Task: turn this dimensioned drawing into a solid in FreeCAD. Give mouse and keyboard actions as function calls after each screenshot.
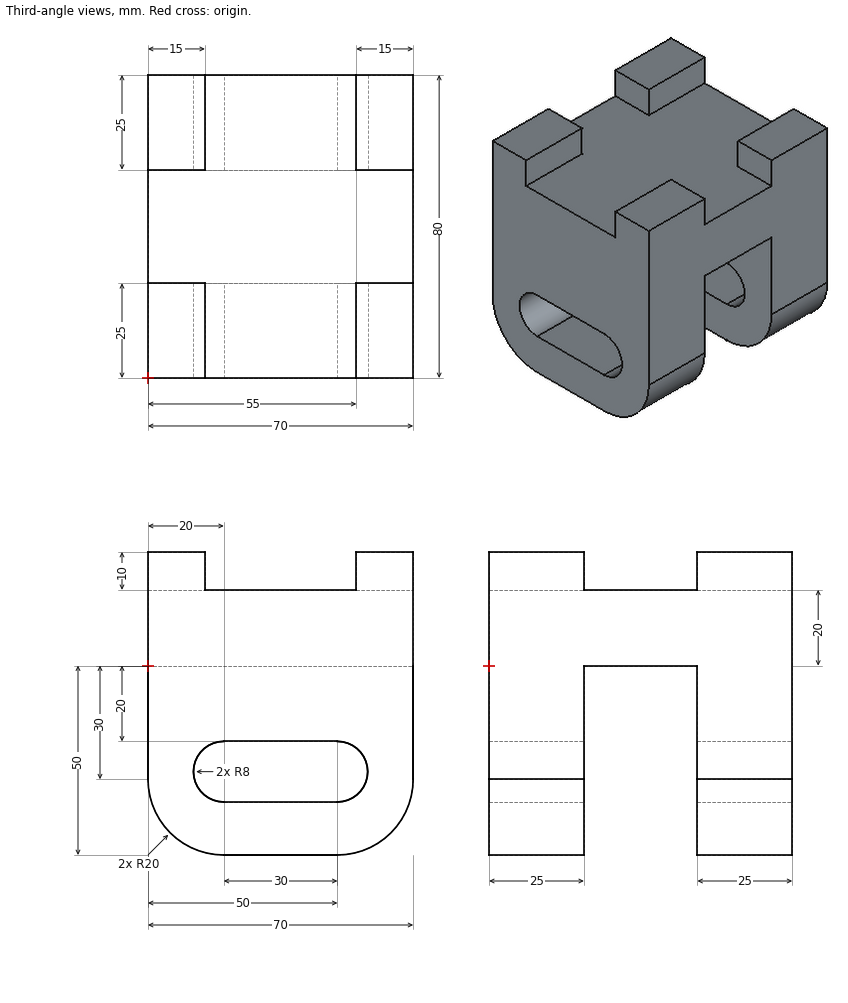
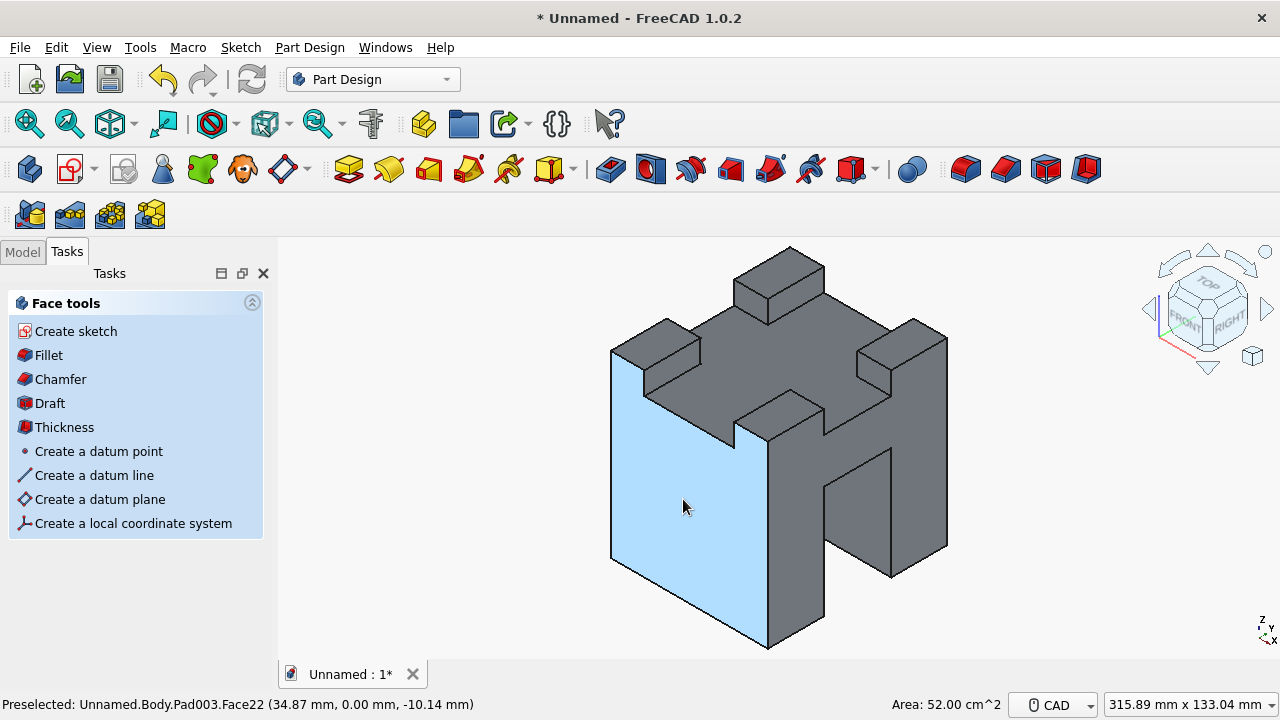
click(70, 170)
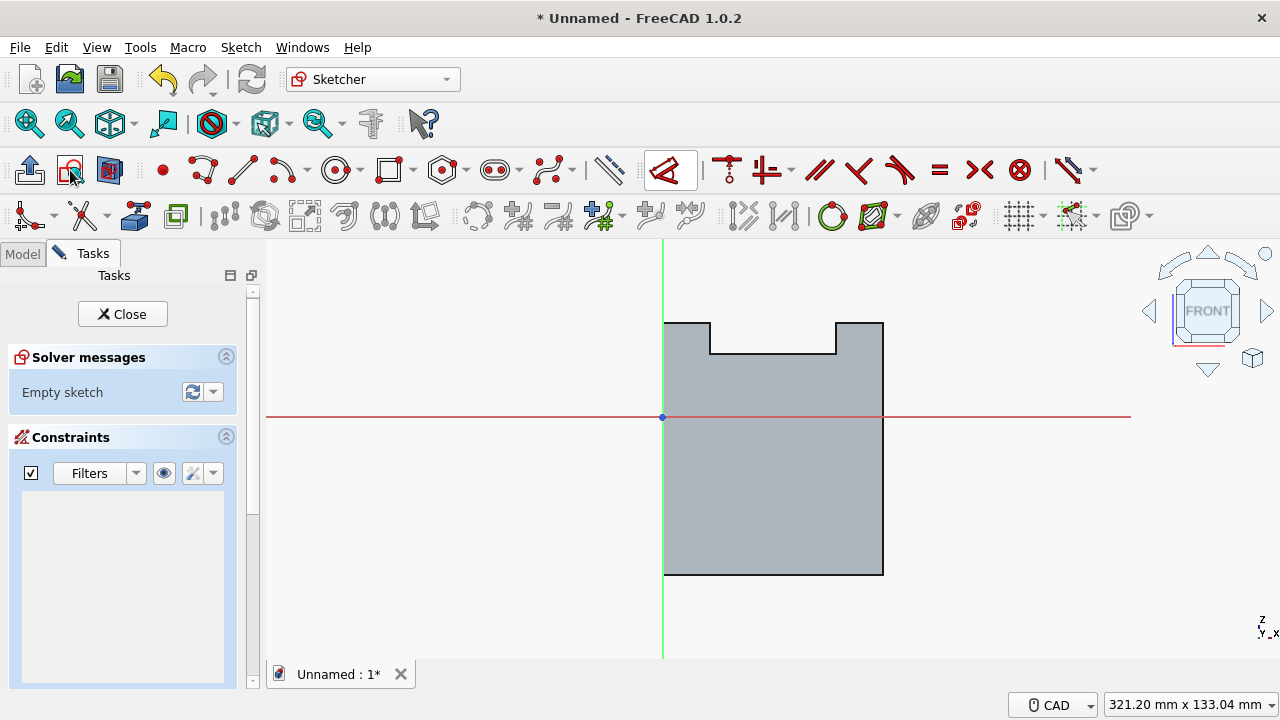
scroll(794, 495, up, 4)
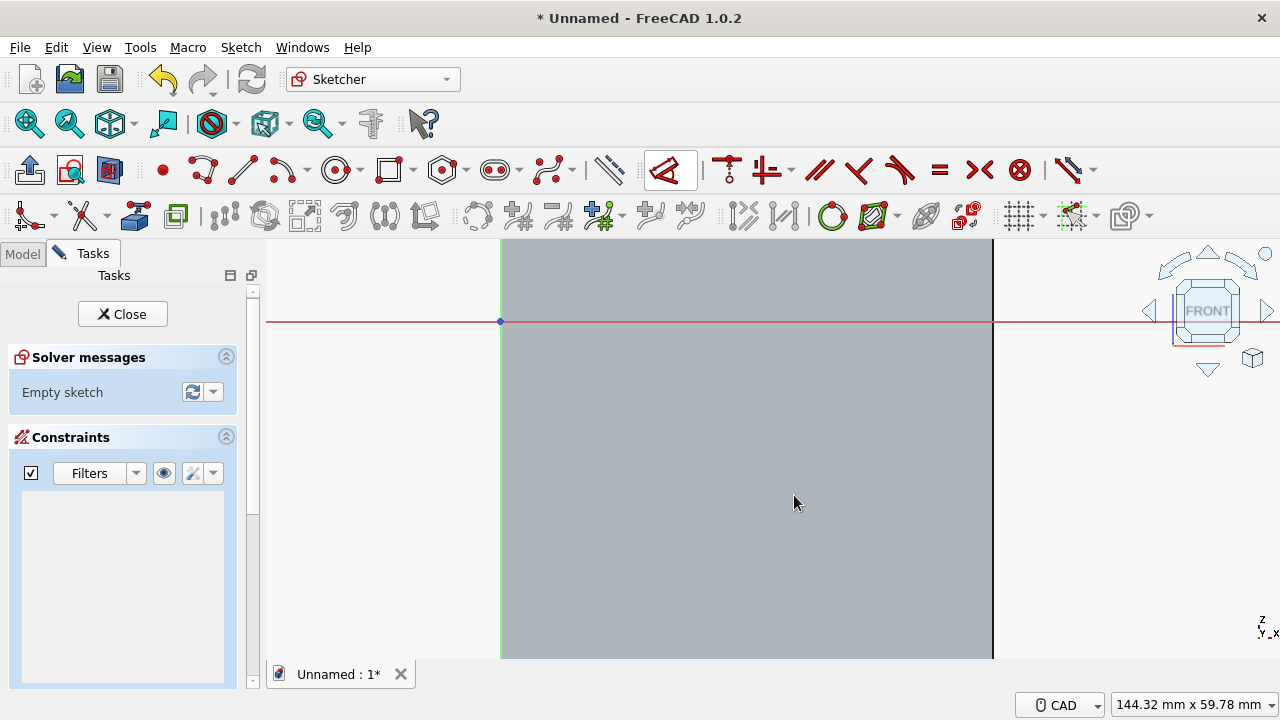
click(496, 170)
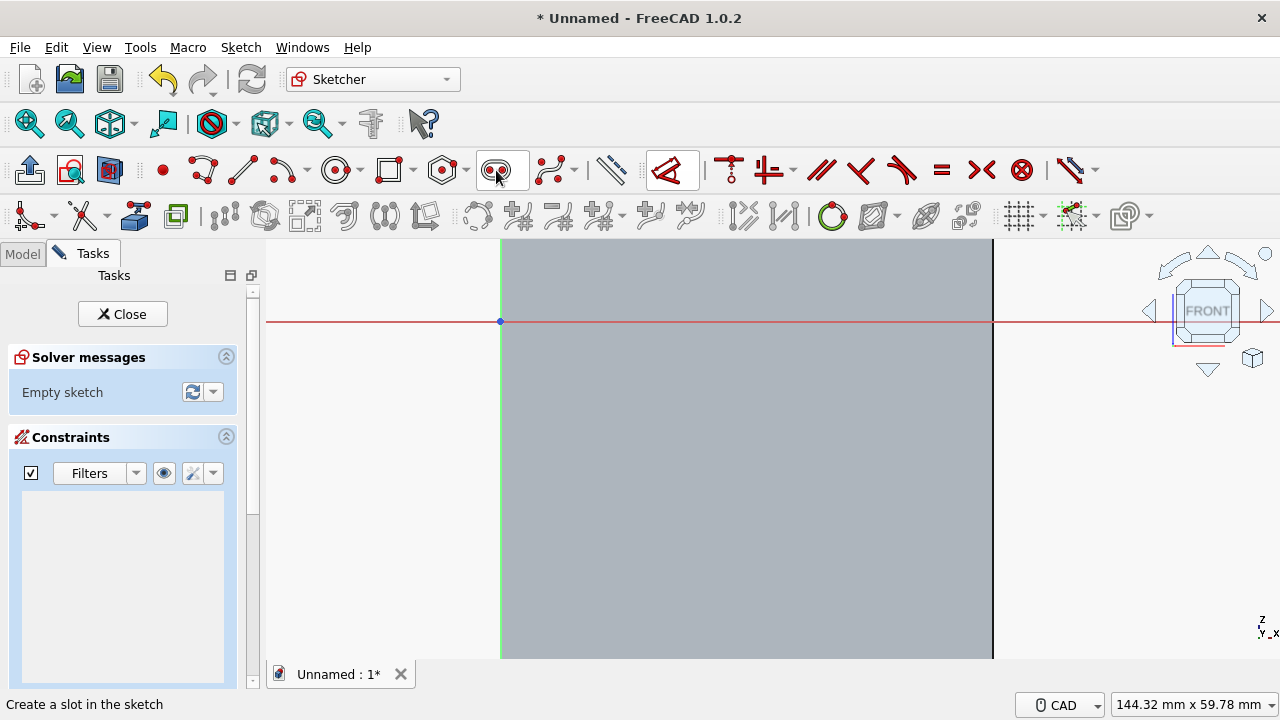
click(641, 518)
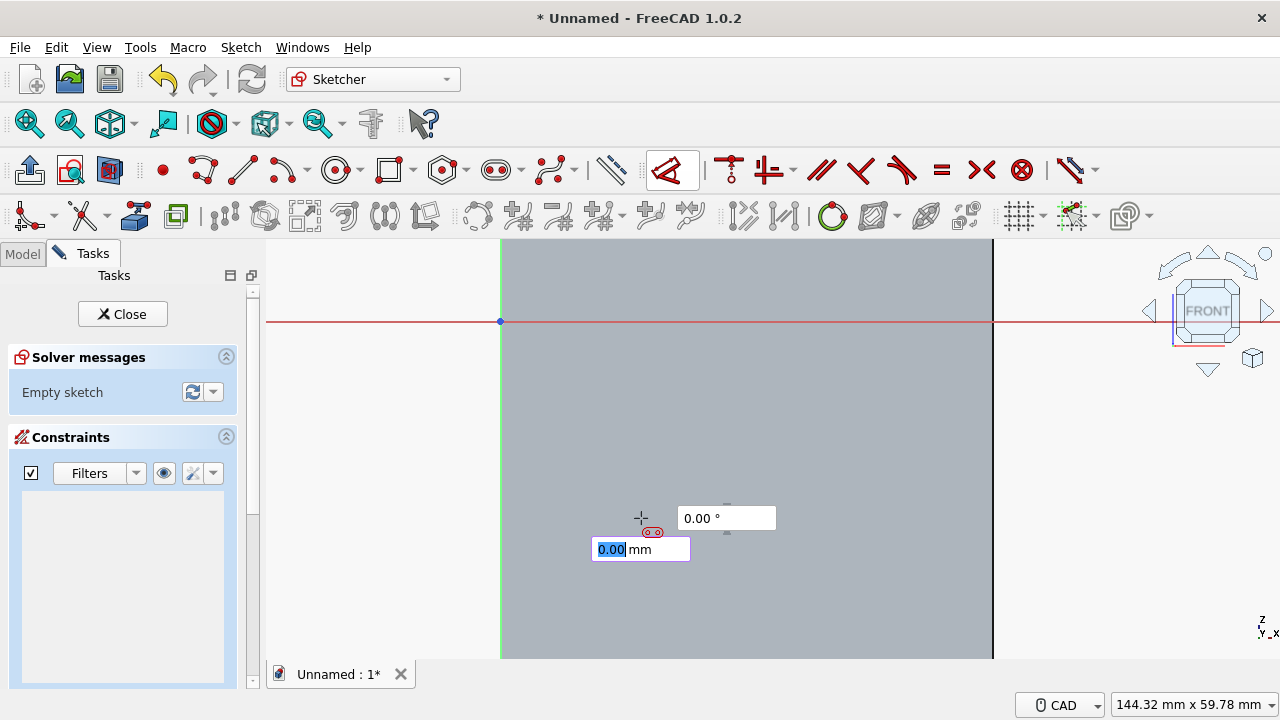
click(852, 518)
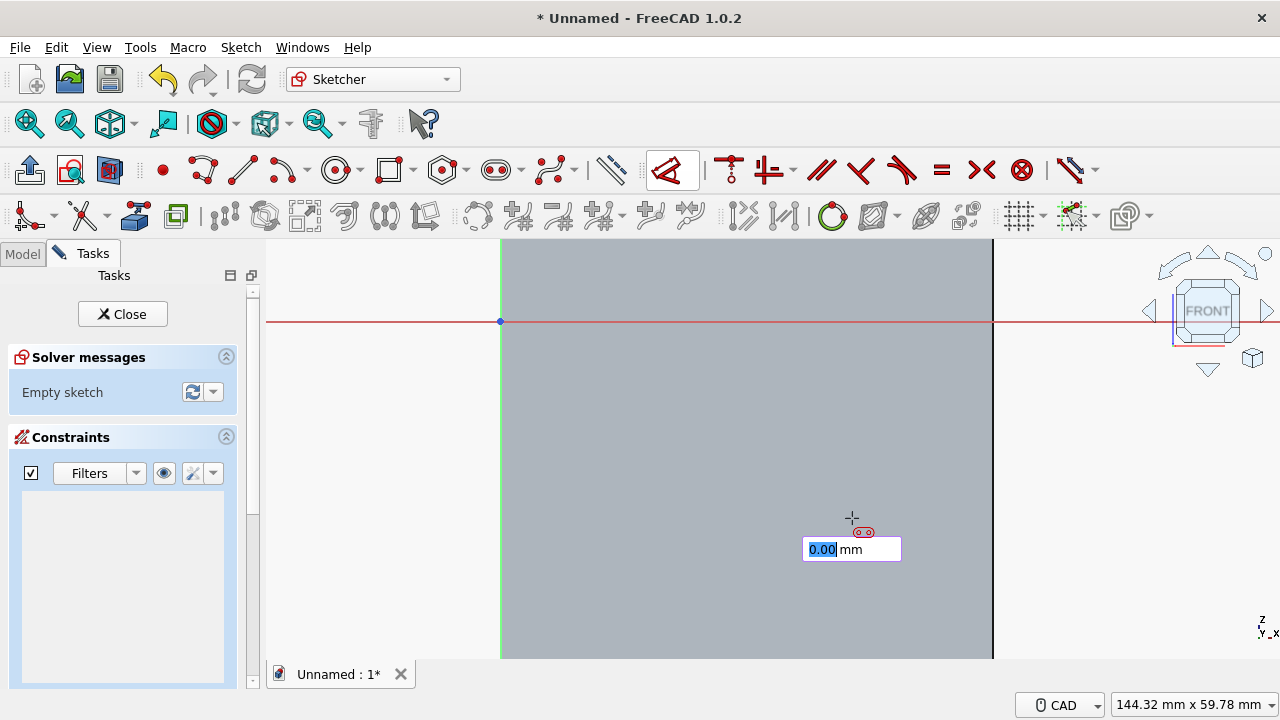
click(747, 462)
key(Escape)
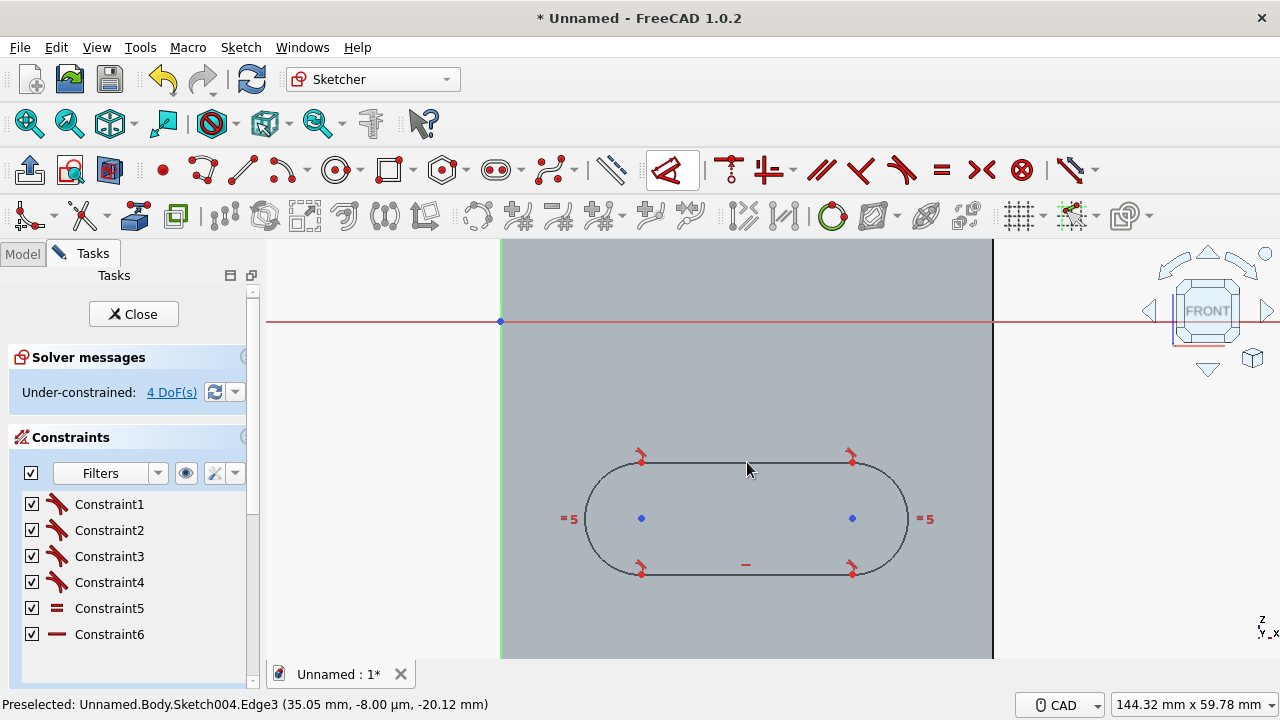
click(596, 486)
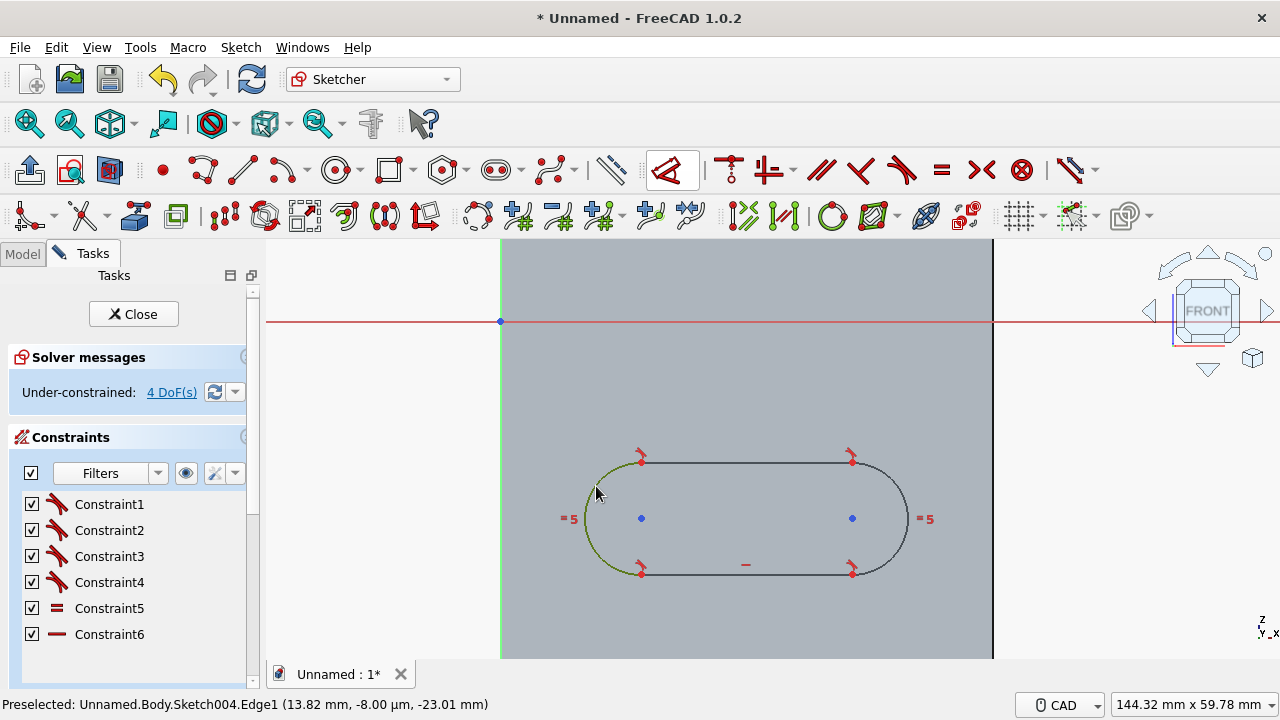
key(k)
key(r)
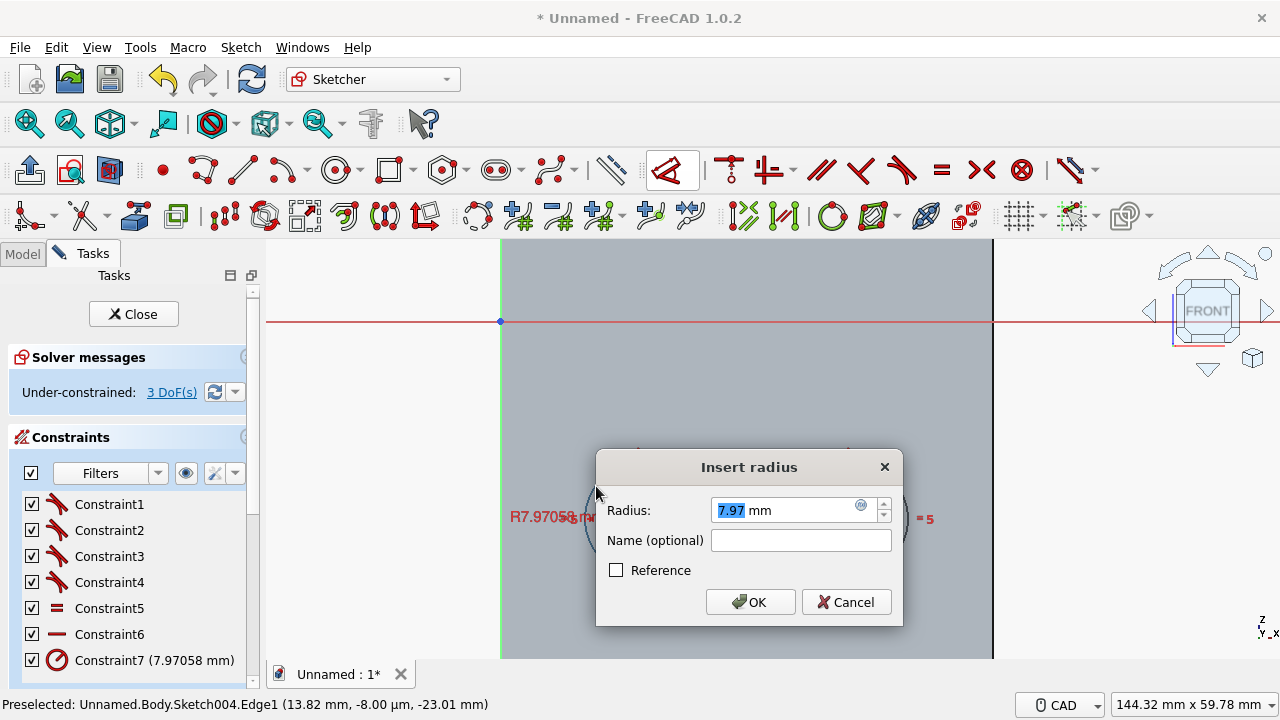
text(8)
key(Return)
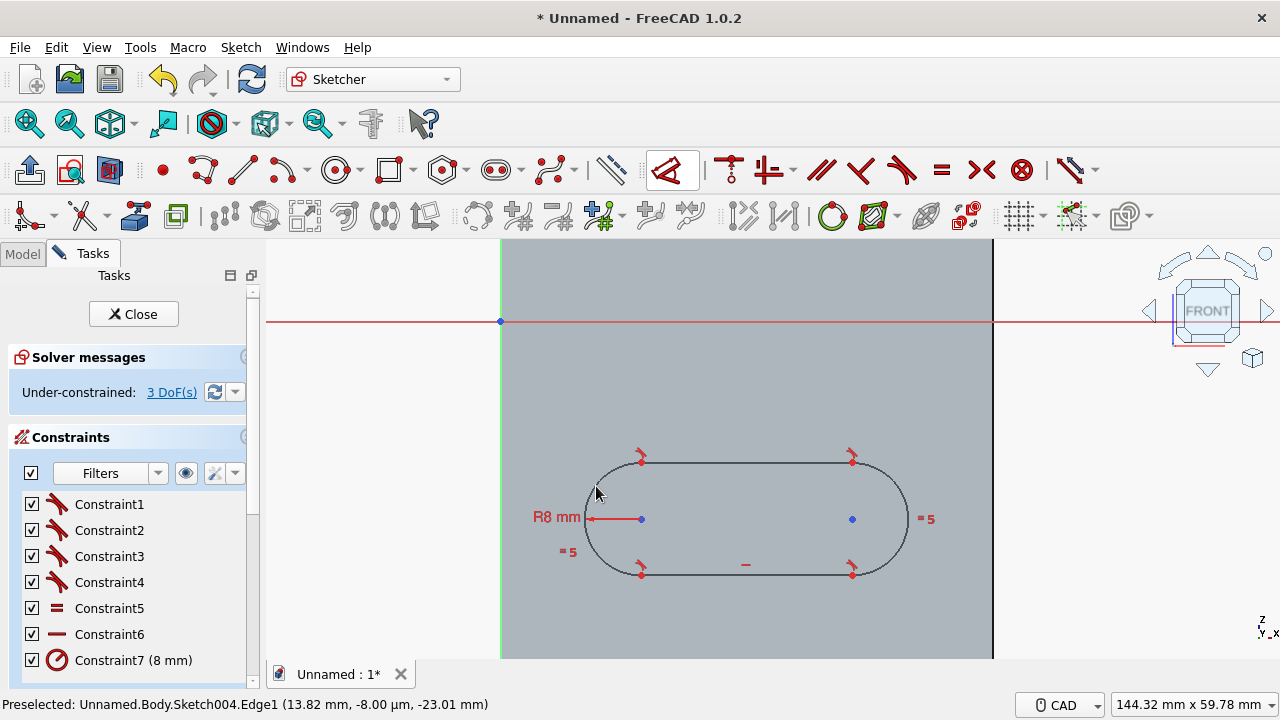
click(704, 463)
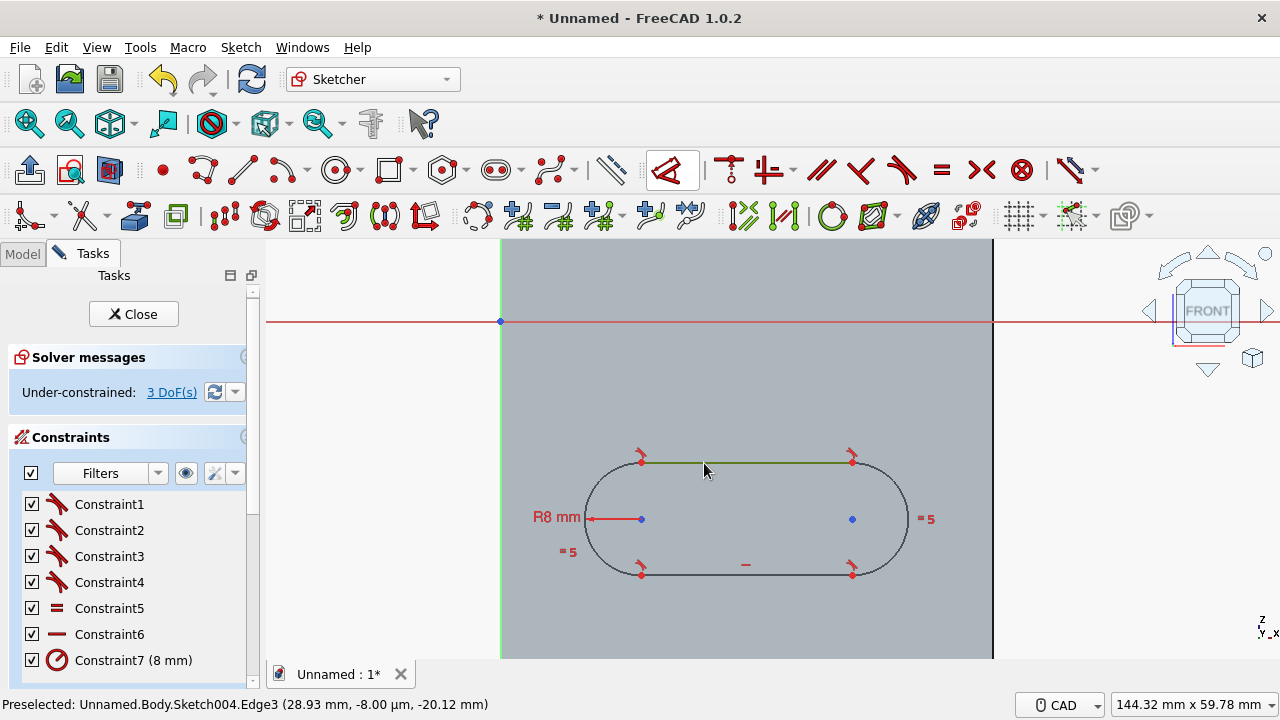
key(l)